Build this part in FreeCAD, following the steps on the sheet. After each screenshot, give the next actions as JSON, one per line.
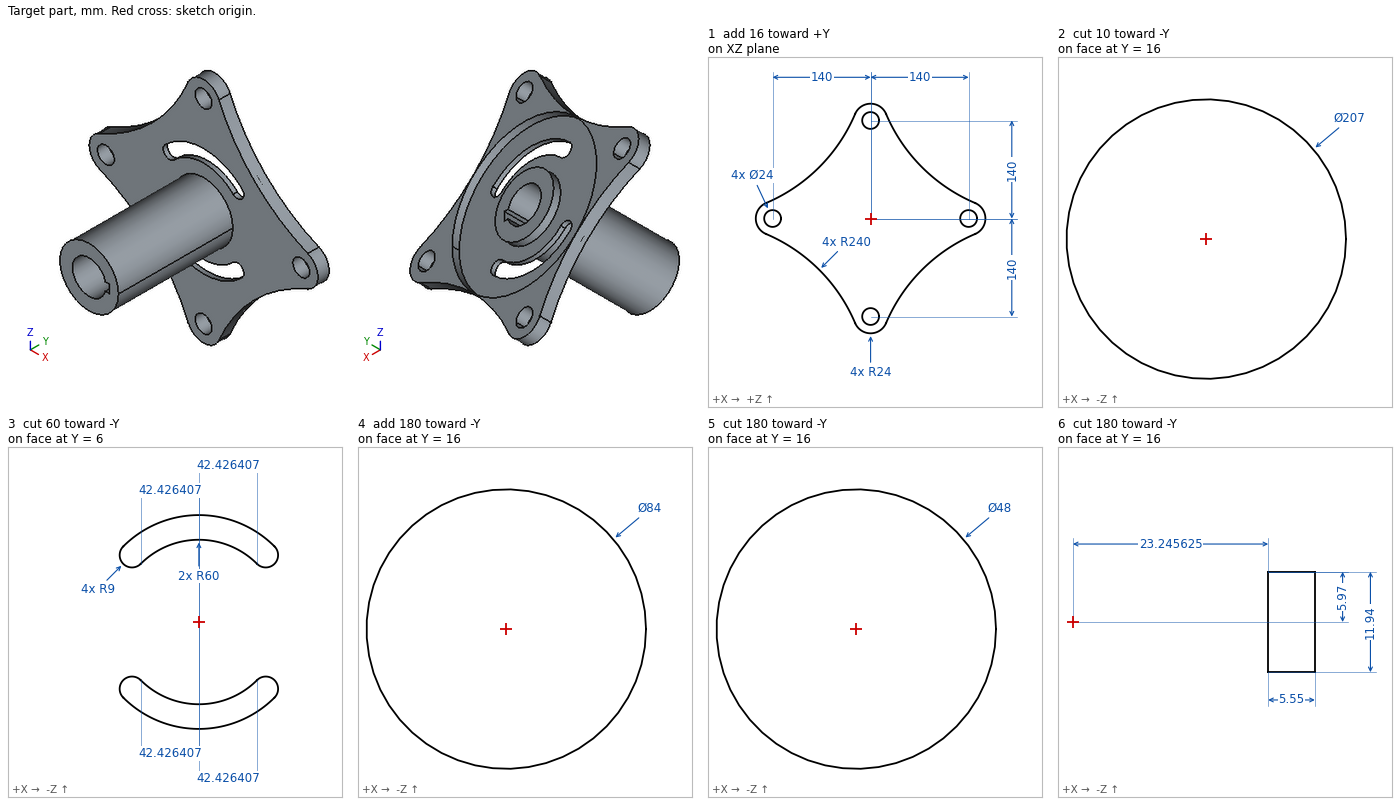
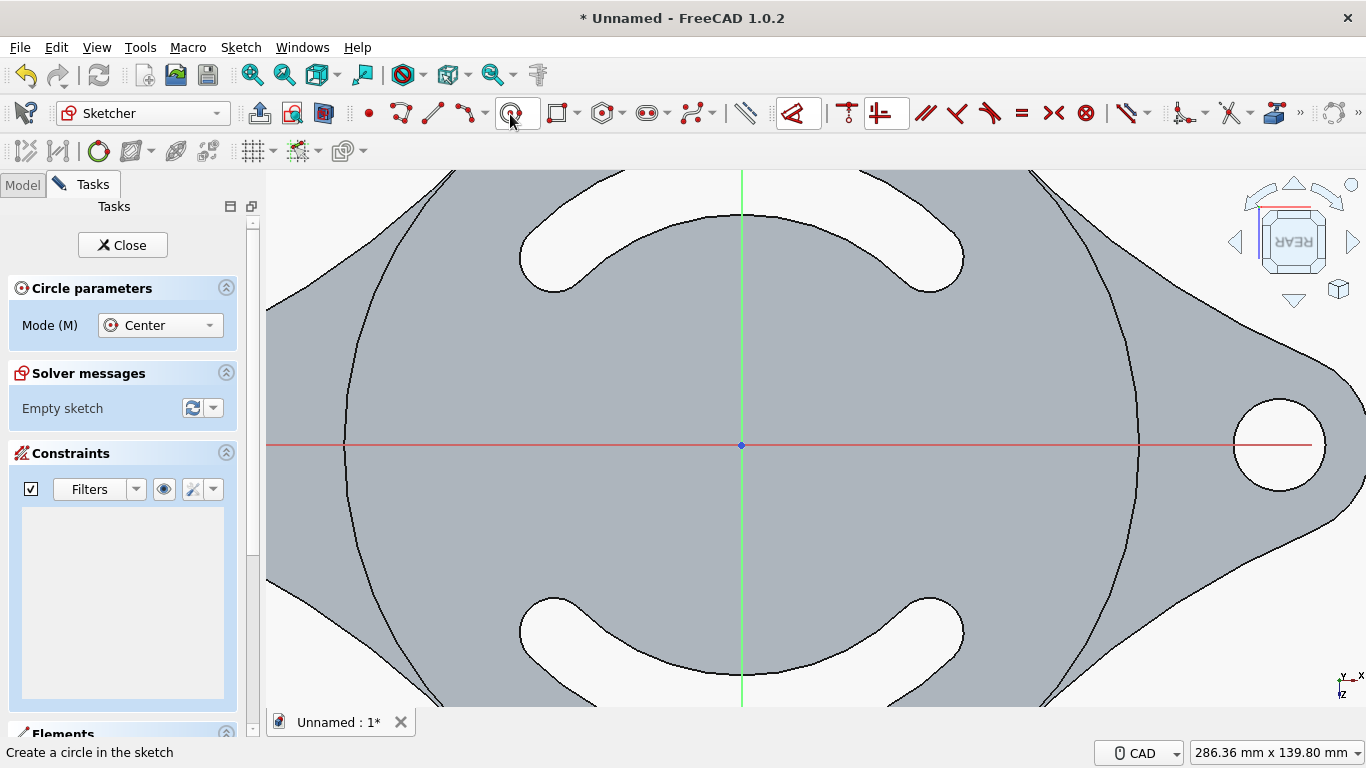
{"action": "left_click", "coordinate": [742, 445]}
{"action": "left_click", "coordinate": [856, 331]}
{"action": "key", "text": "Escape"}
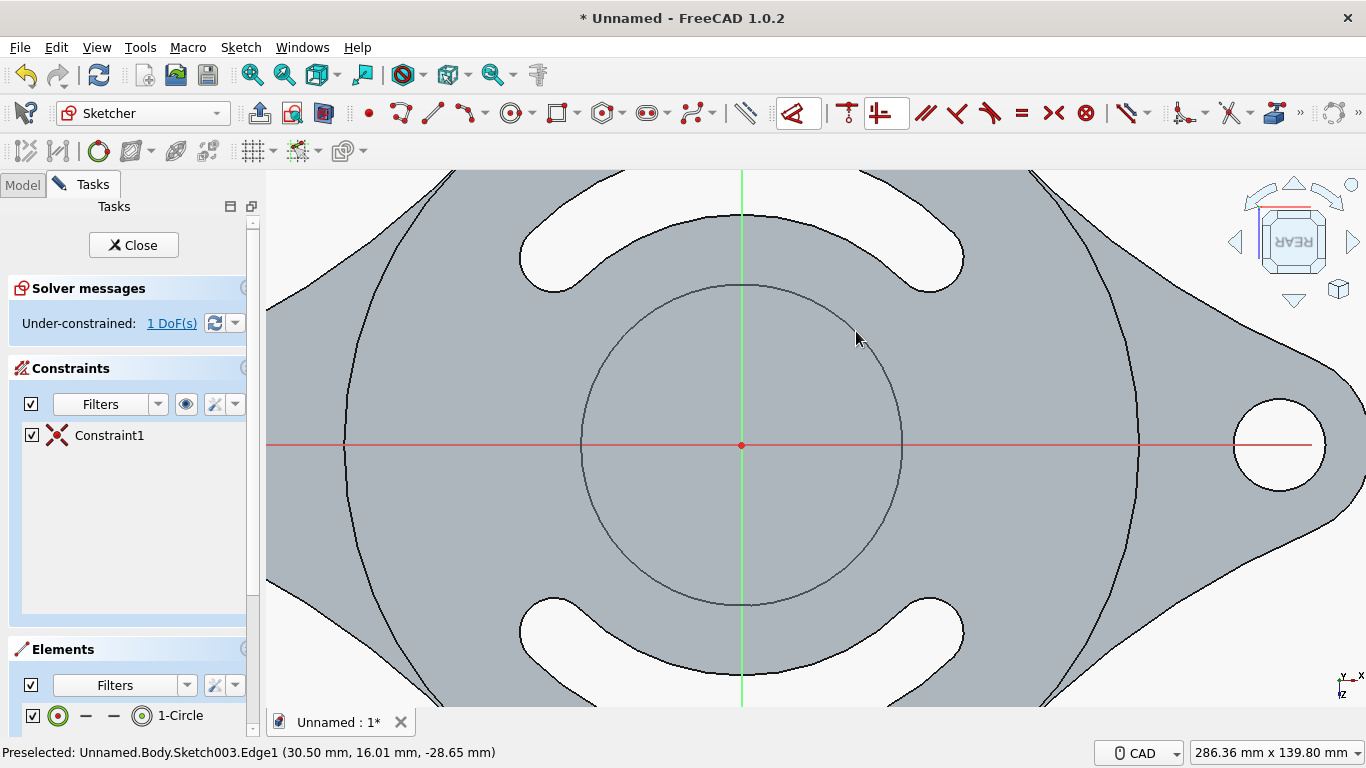
{"action": "left_click", "coordinate": [855, 331]}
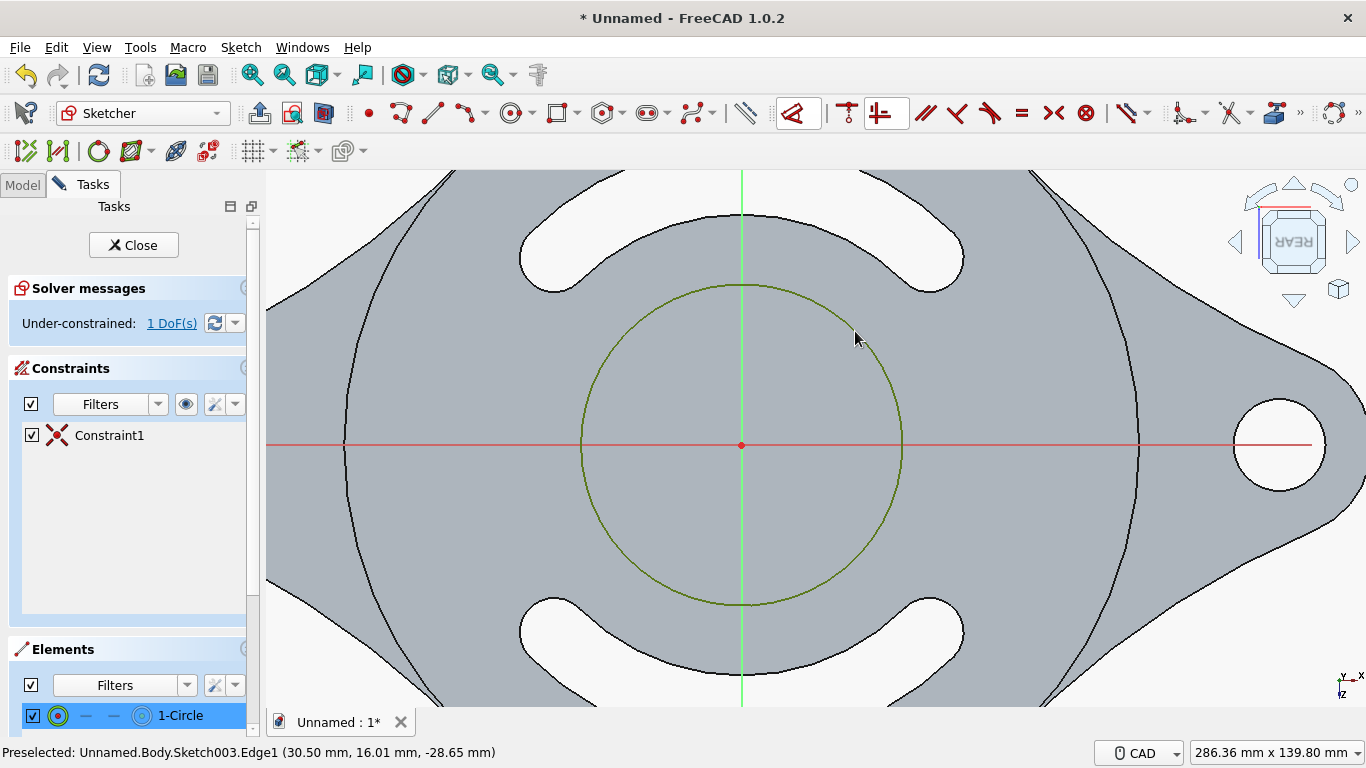
{"action": "key", "text": "k o"}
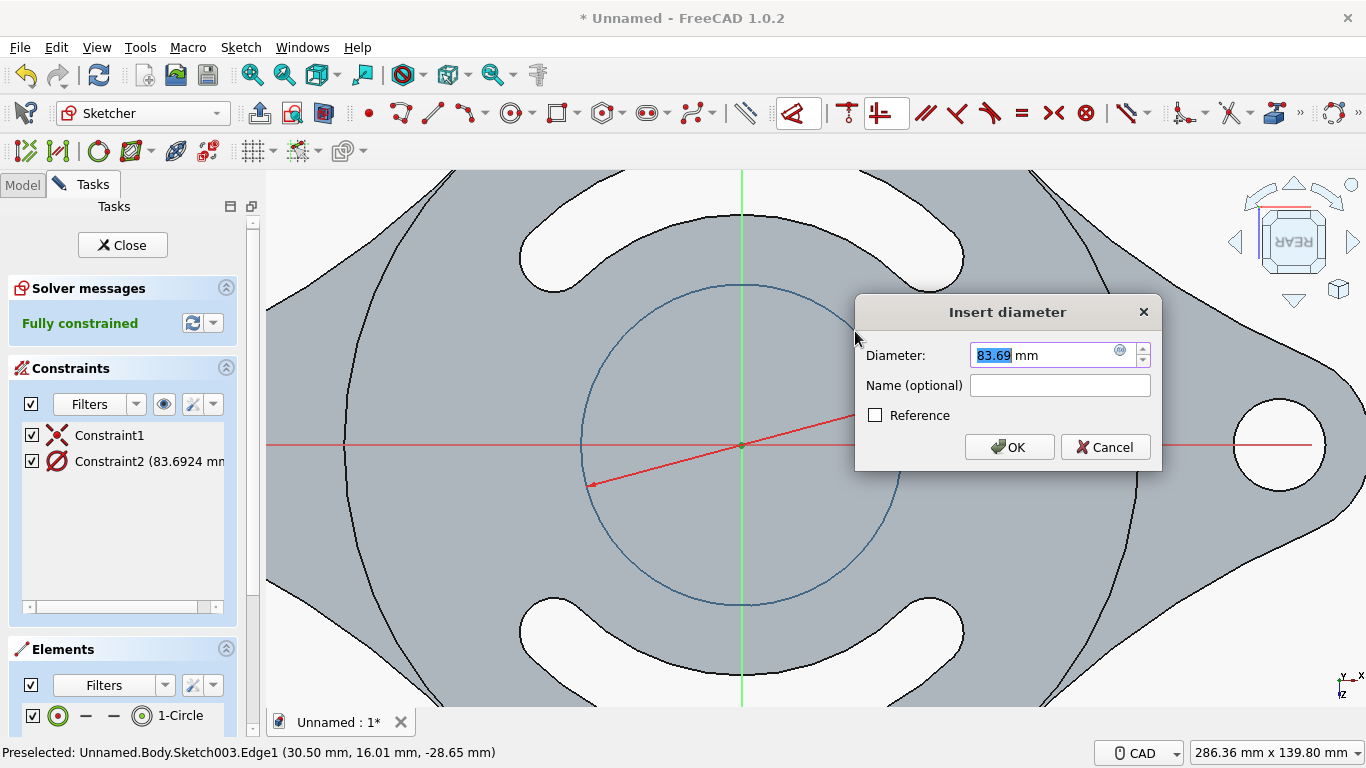
{"action": "type", "text": "84"}
{"action": "key", "text": "Return"}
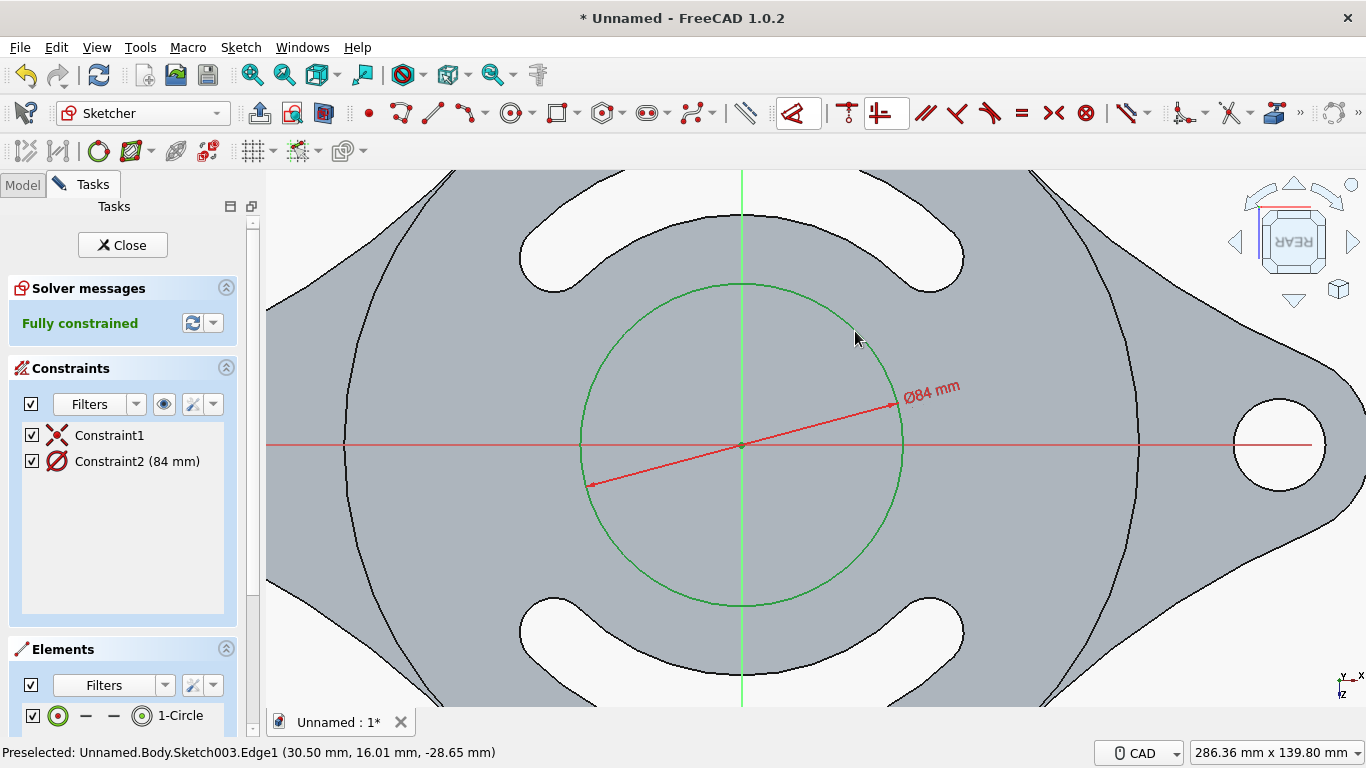
{"action": "left_click", "coordinate": [123, 245]}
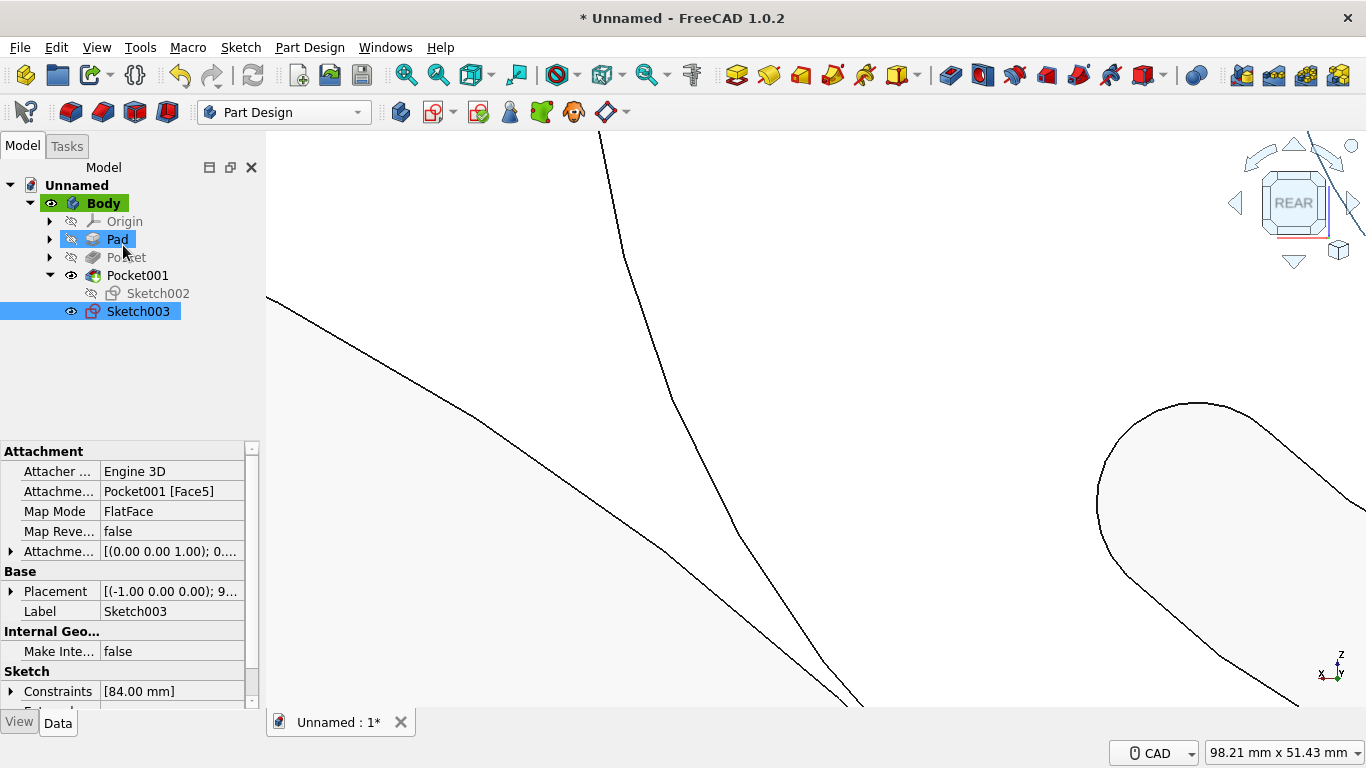
{"action": "left_click", "coordinate": [738, 76]}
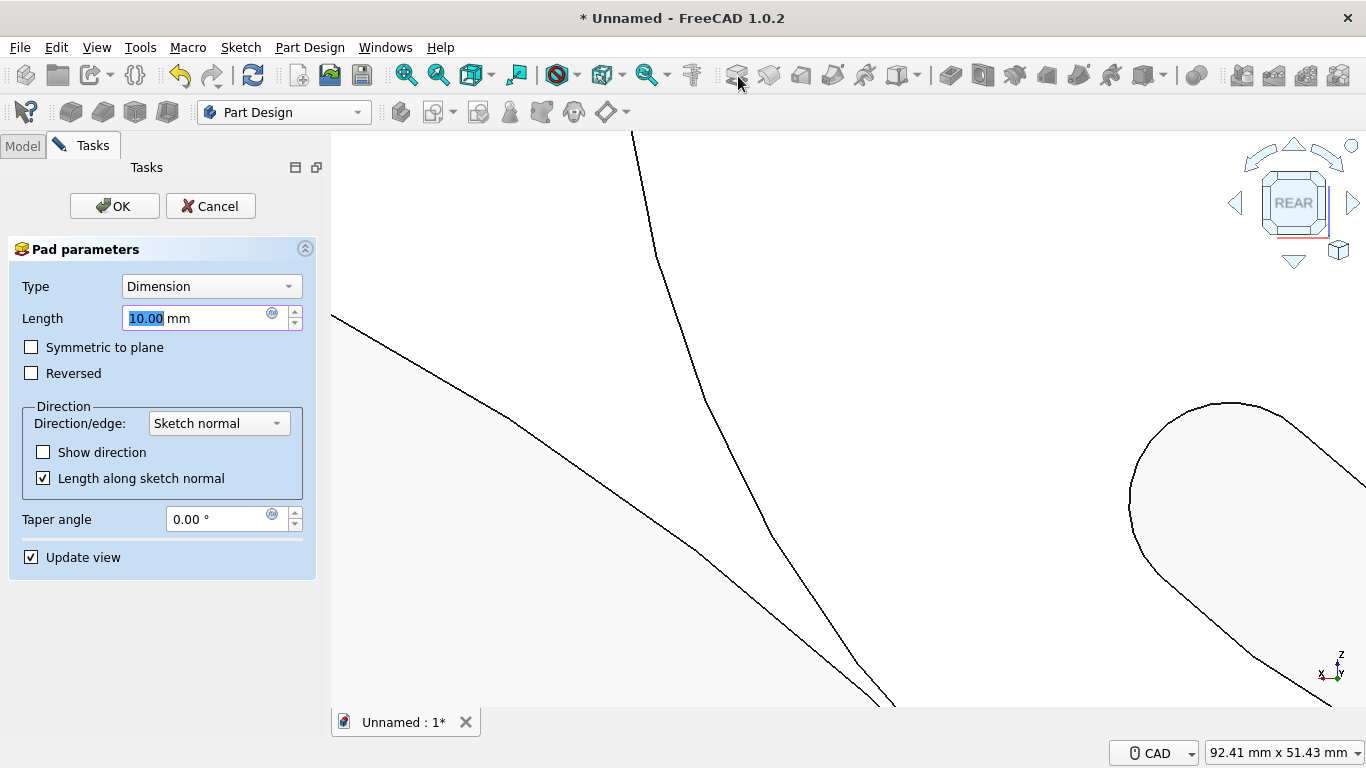
{"action": "type", "text": "180"}
{"action": "key", "text": "Tab"}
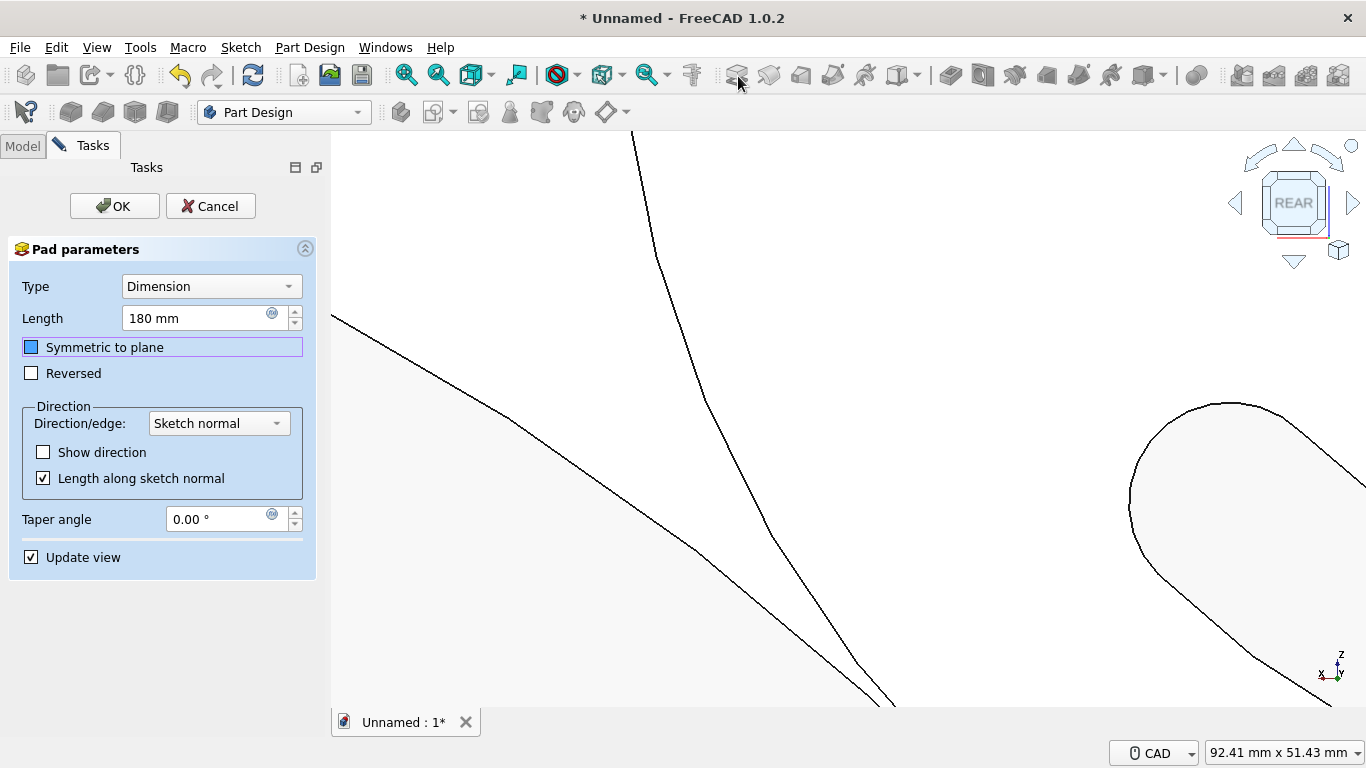
{"action": "left_click", "coordinate": [30, 373]}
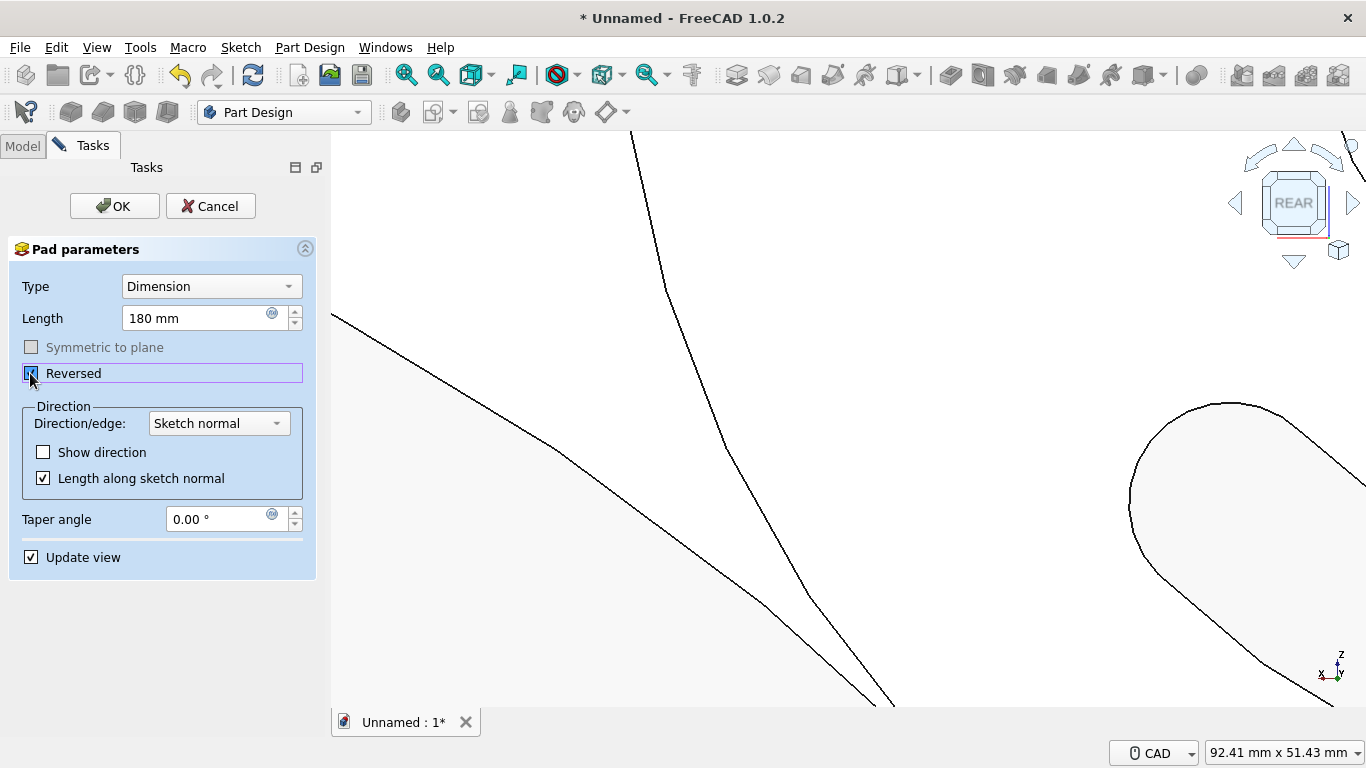
{"action": "left_click", "coordinate": [115, 206]}